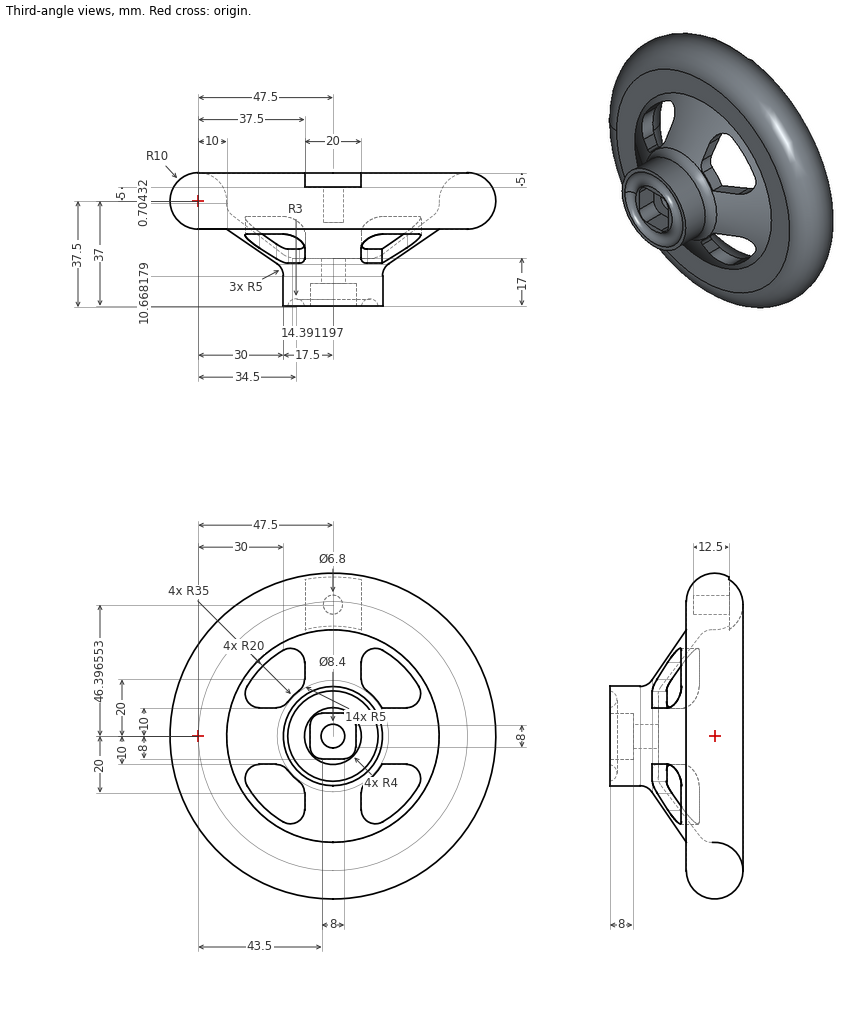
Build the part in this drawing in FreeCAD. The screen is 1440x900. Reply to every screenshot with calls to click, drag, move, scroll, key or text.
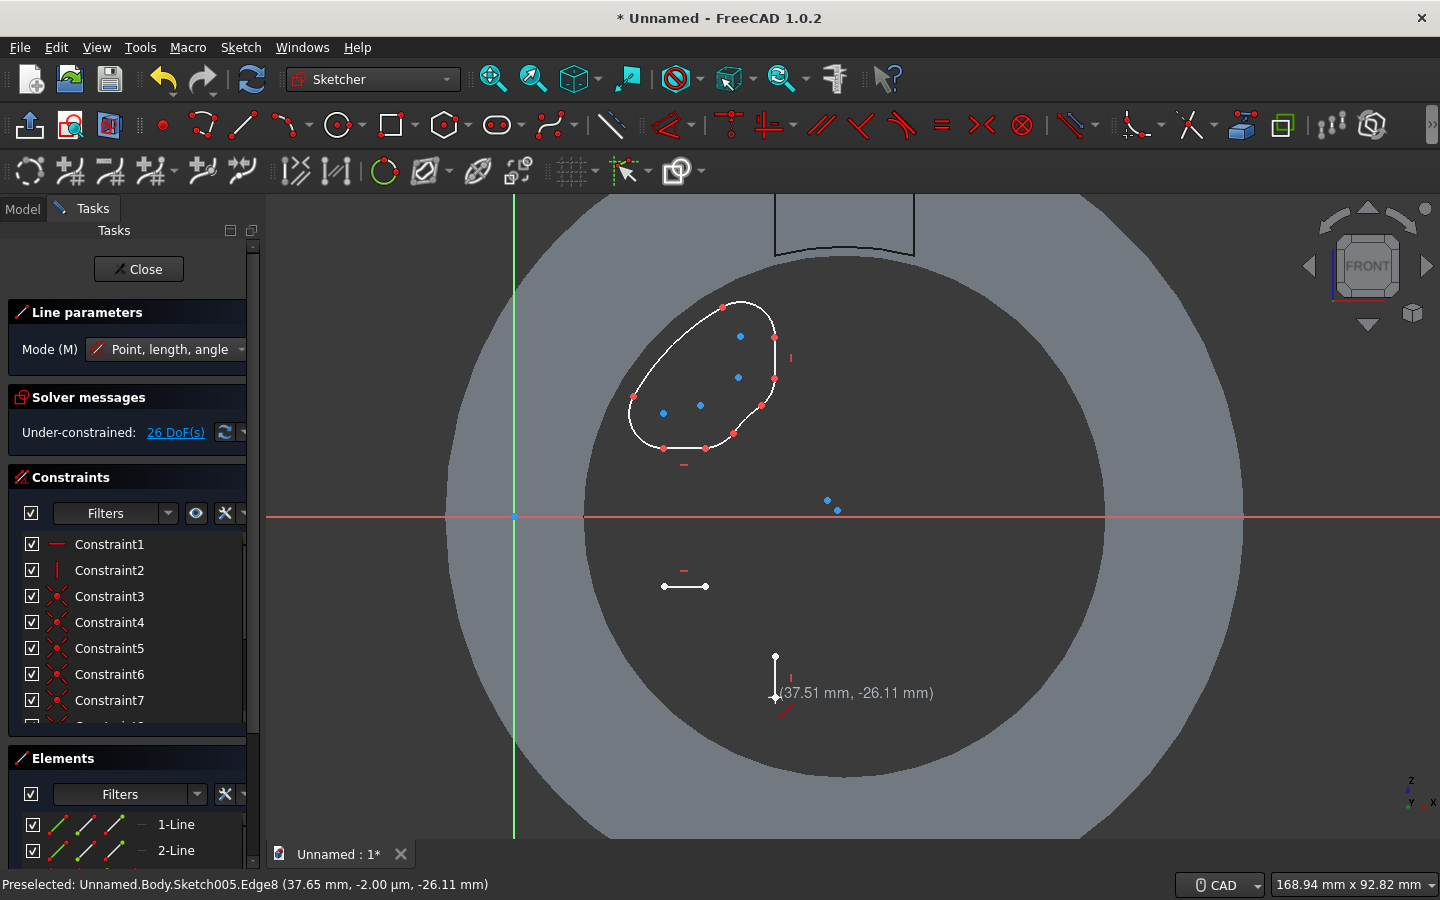
click(284, 126)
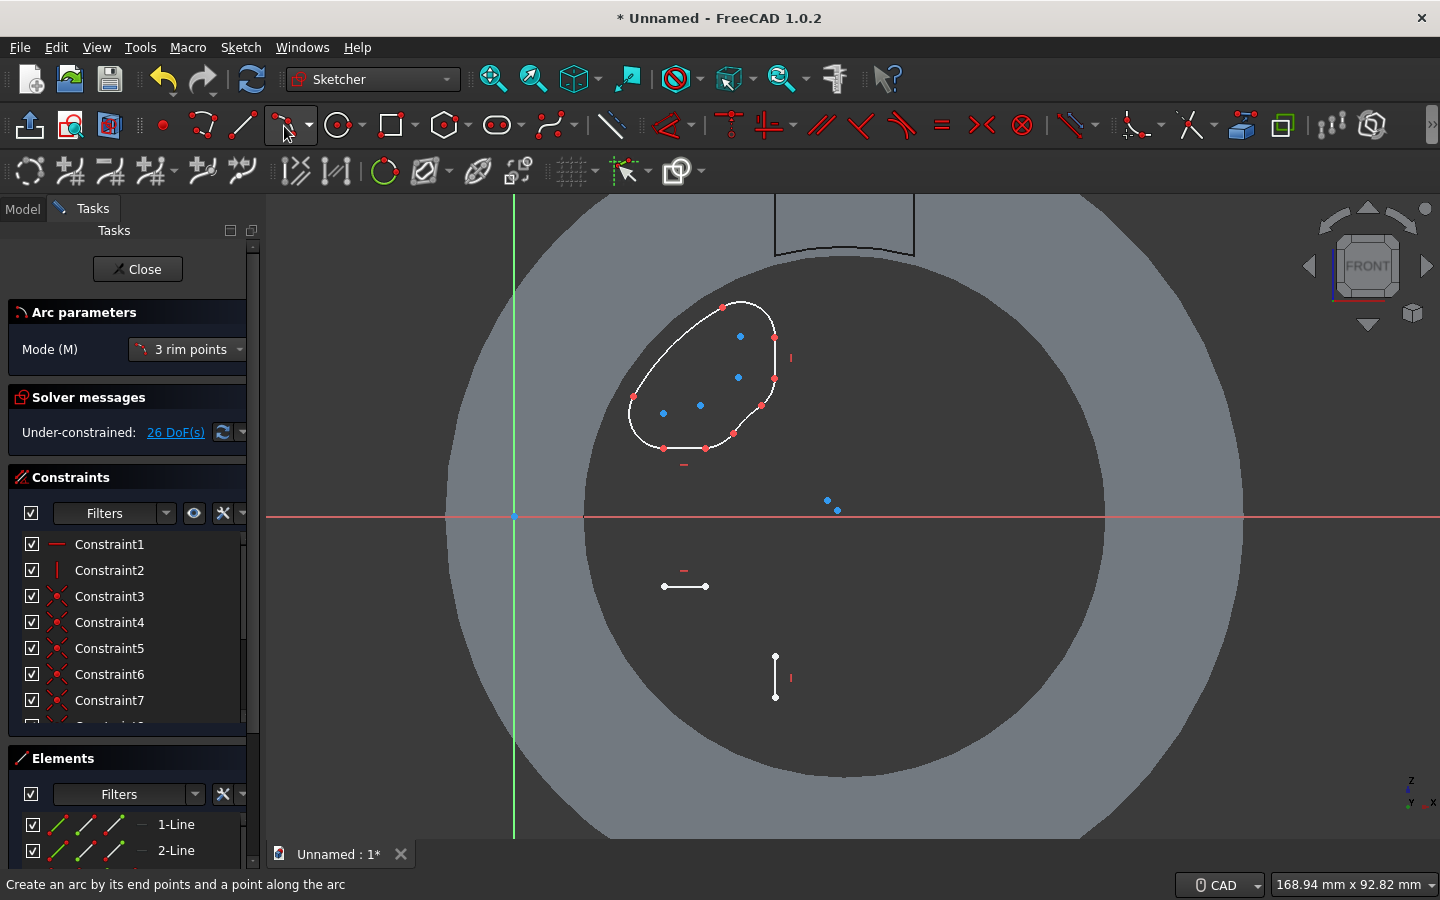
click(705, 587)
click(733, 600)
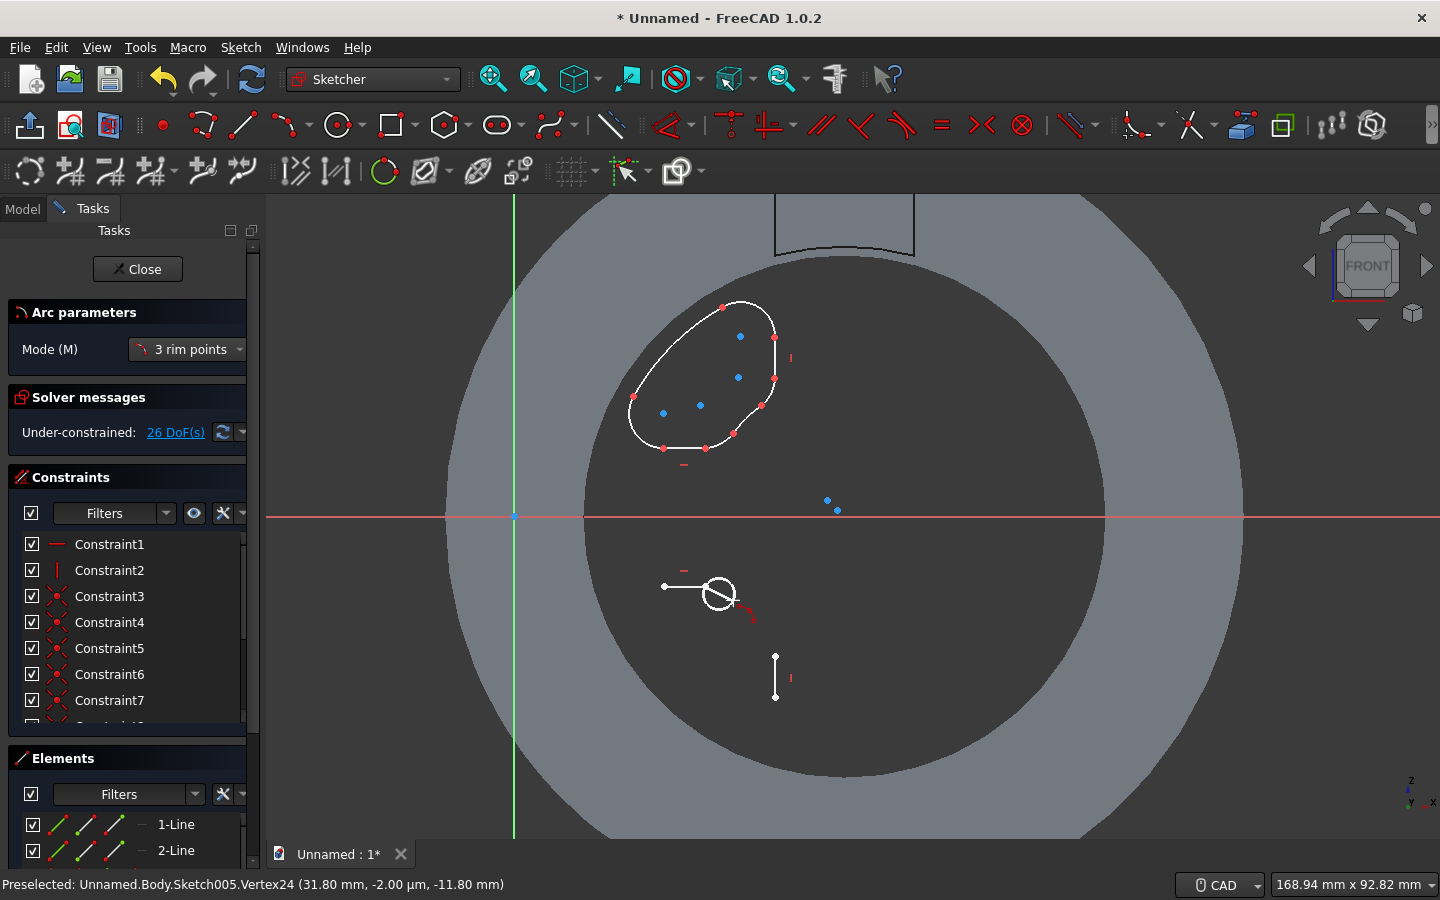
scroll(721, 590, up, 8)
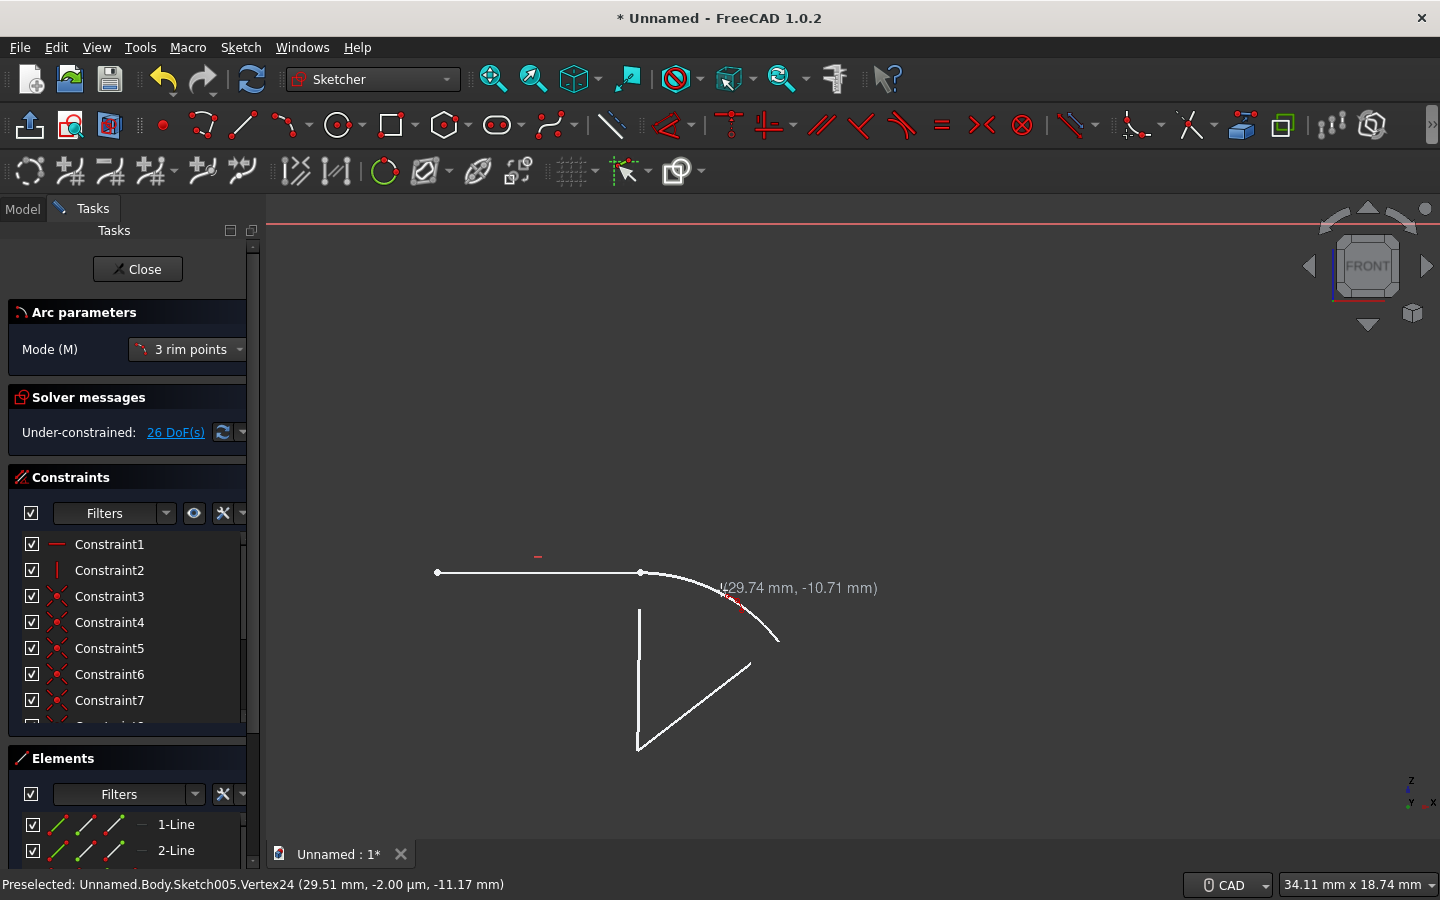
click(719, 586)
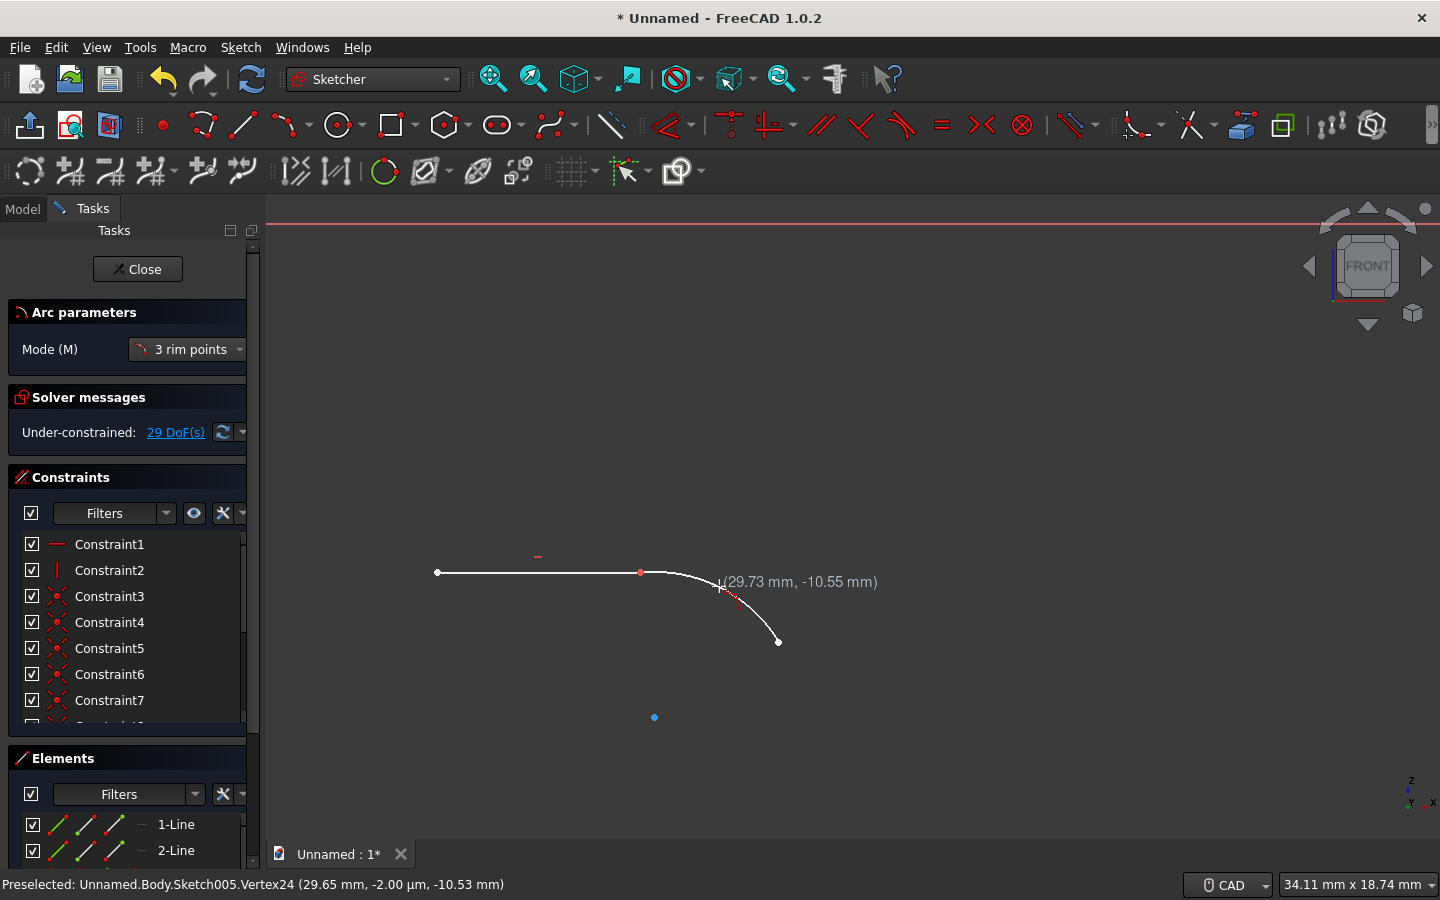
scroll(721, 591, down, 8)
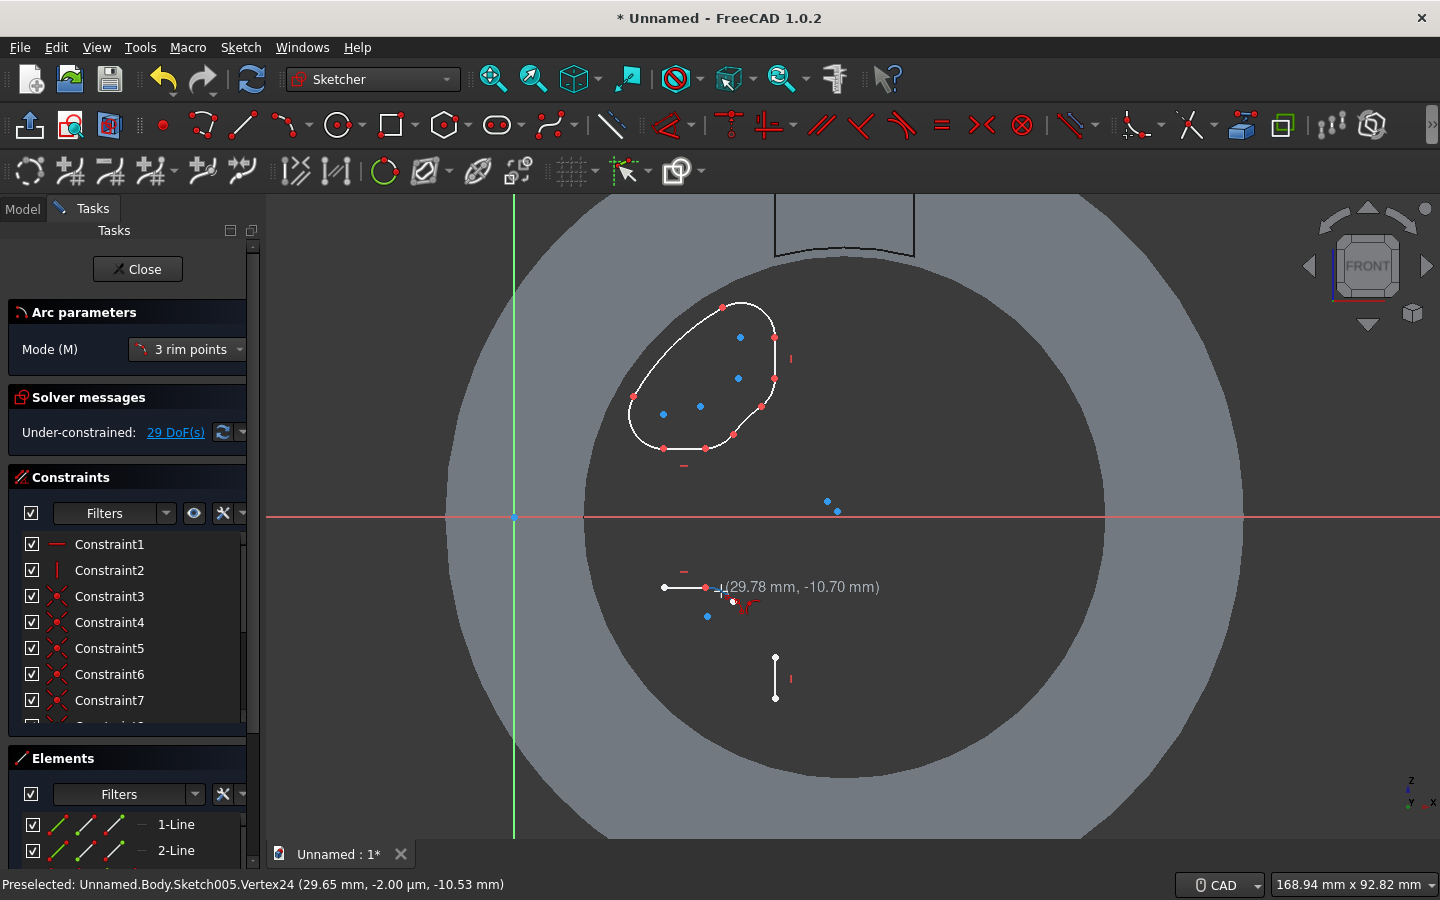
click(733, 602)
click(761, 629)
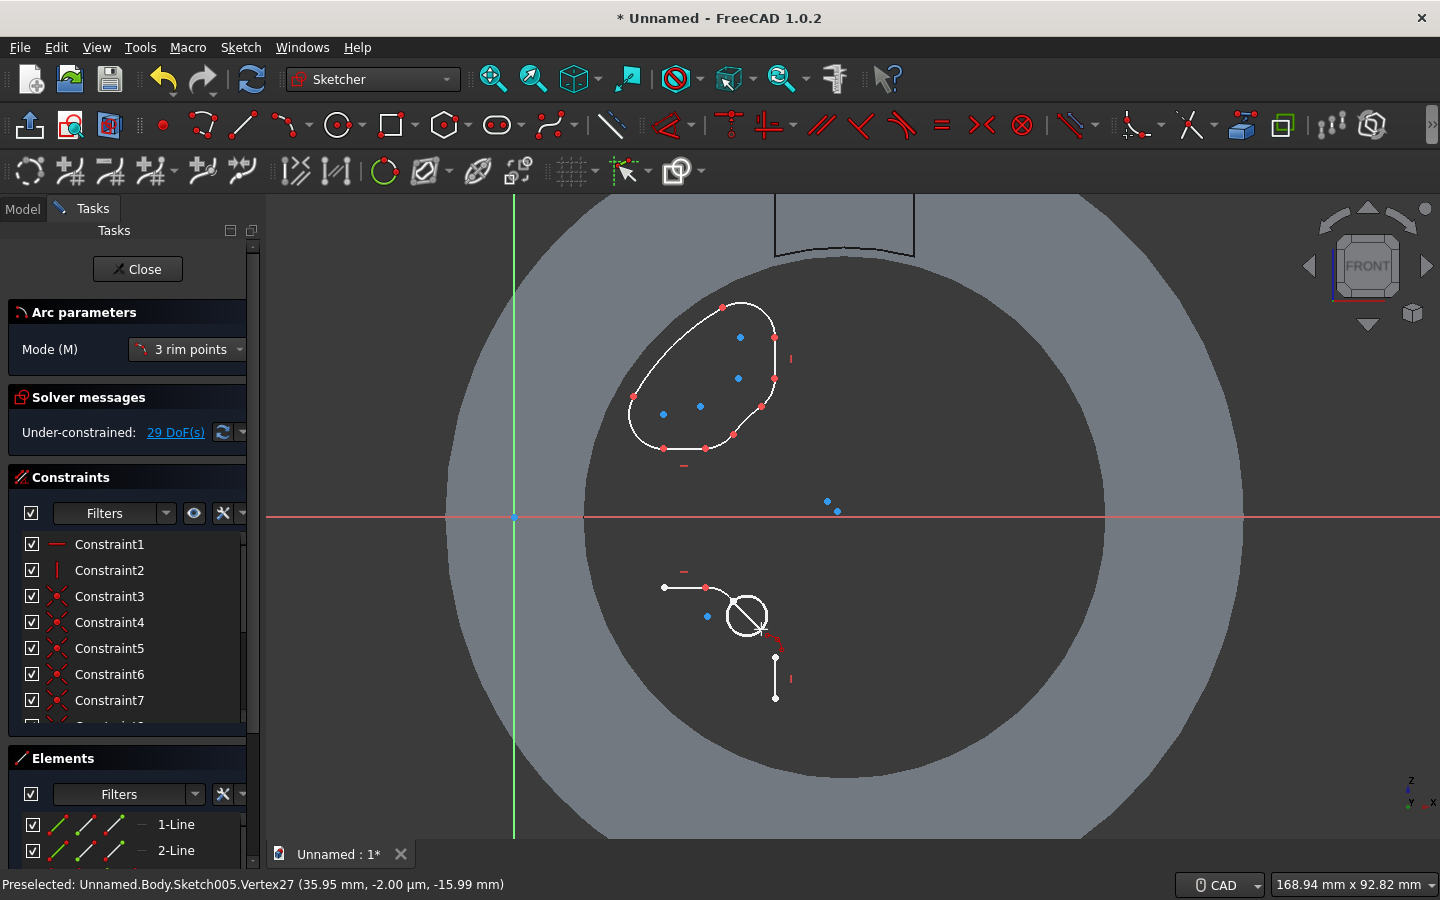
scroll(746, 616, up, 13)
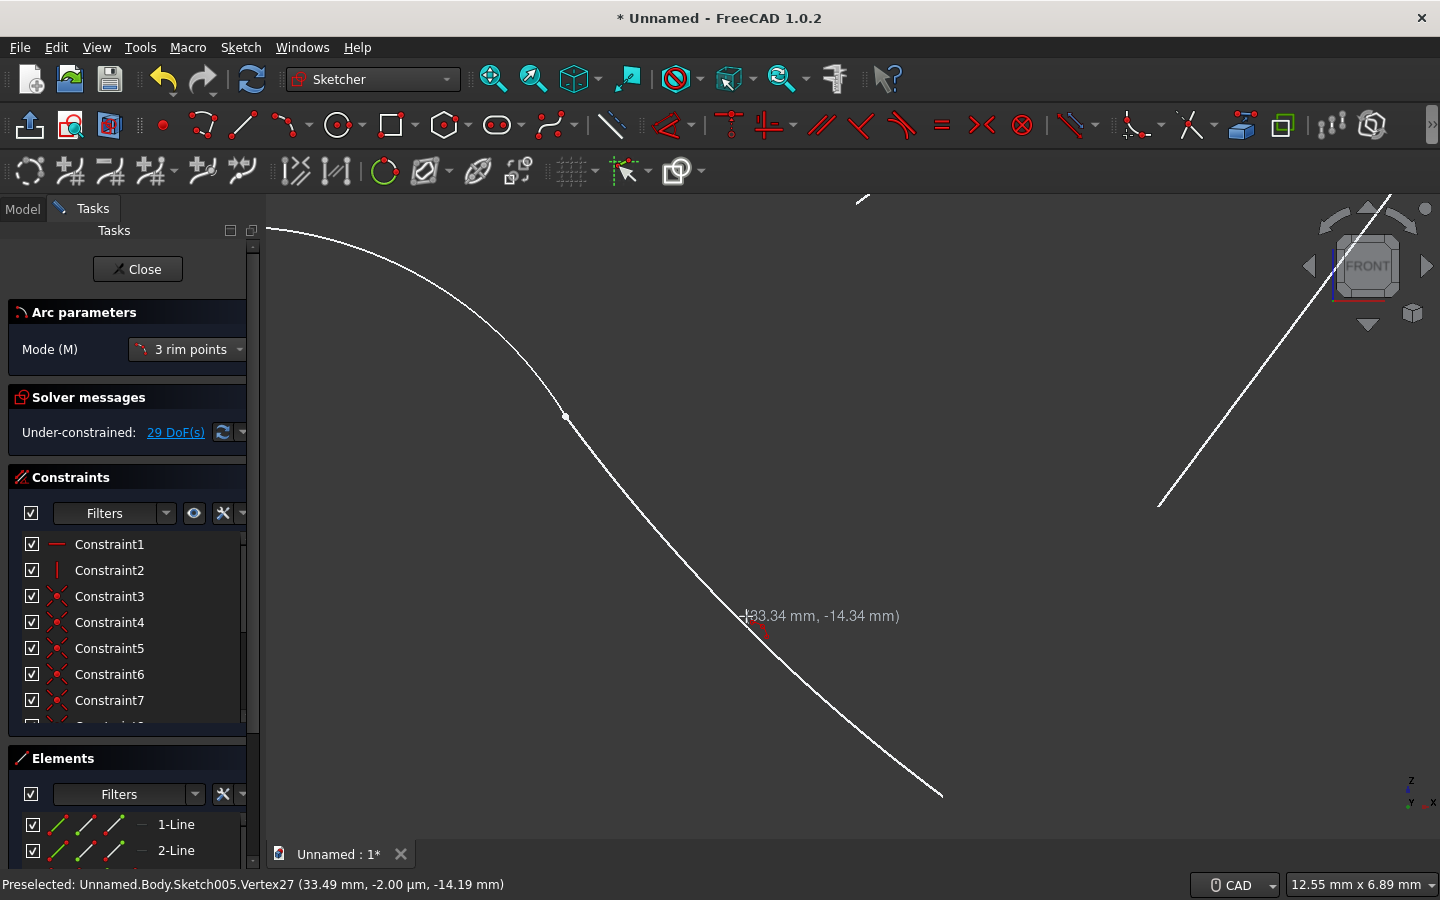
click(743, 603)